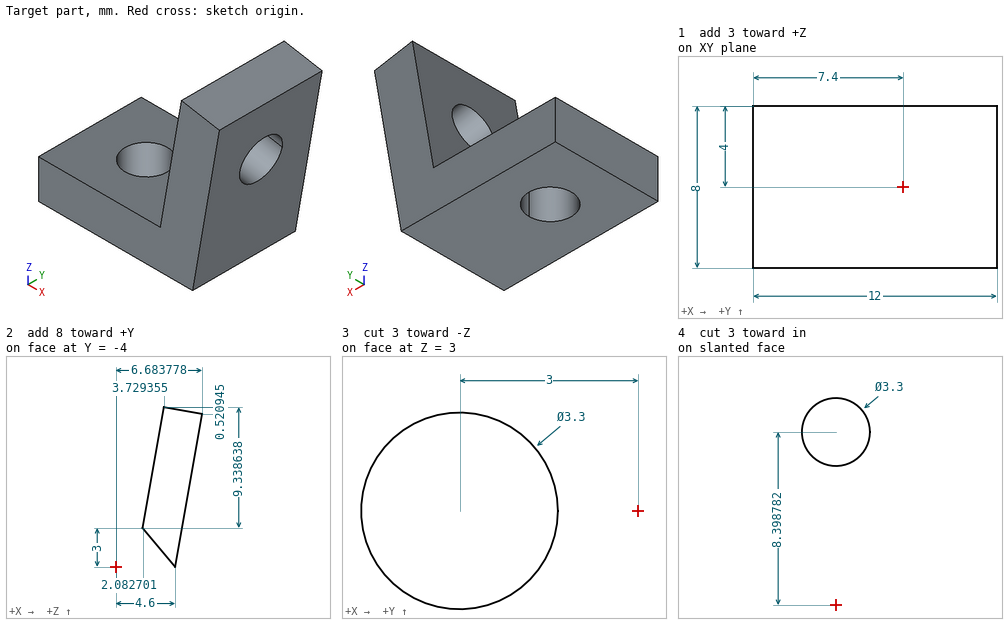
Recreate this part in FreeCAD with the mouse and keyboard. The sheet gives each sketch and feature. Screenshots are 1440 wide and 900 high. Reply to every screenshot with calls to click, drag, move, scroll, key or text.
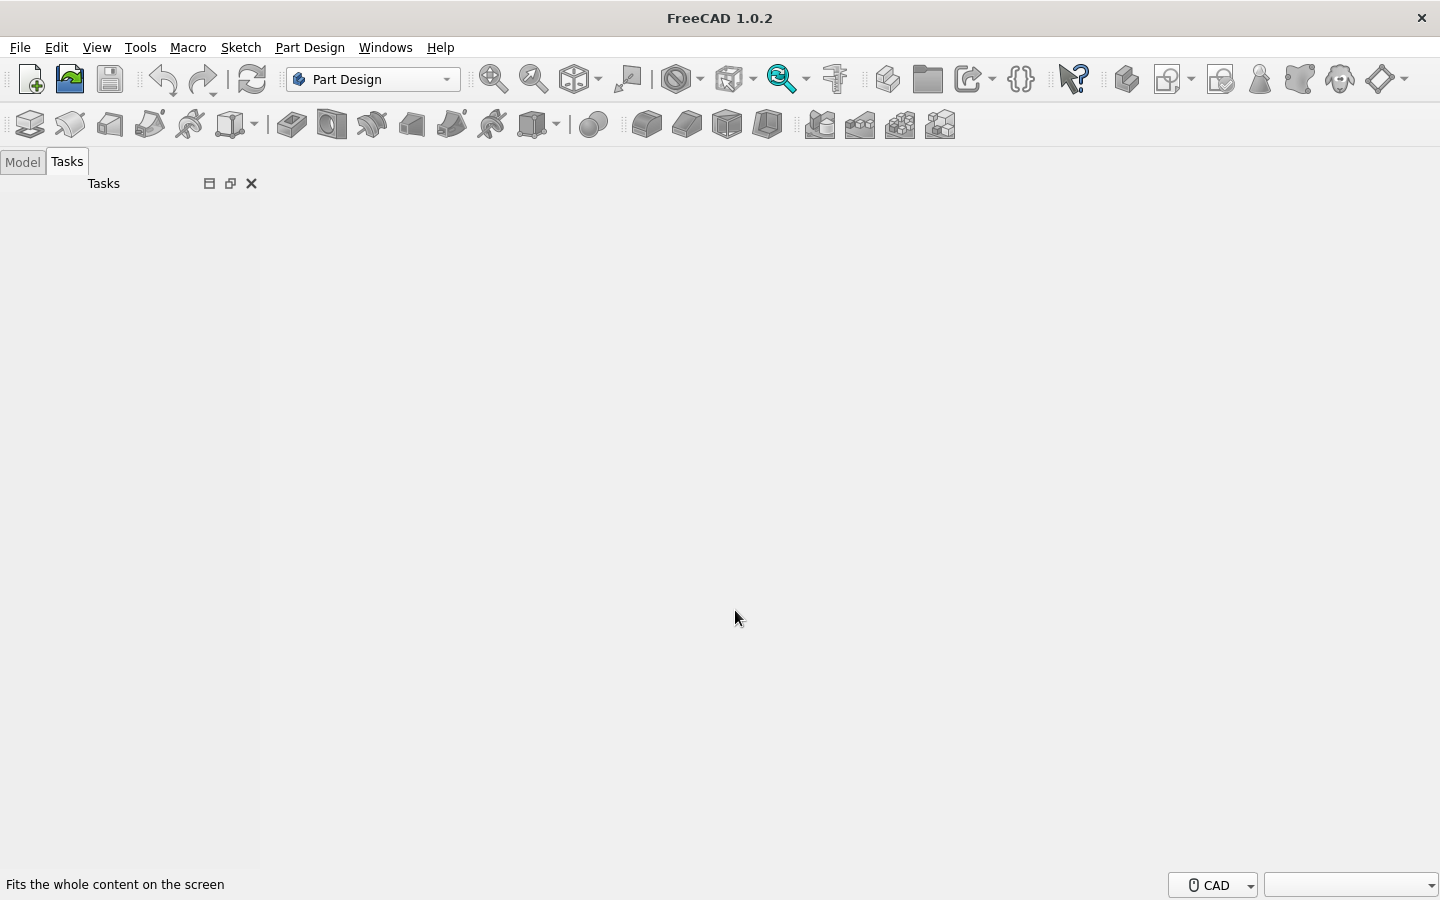
key(ctrl+n)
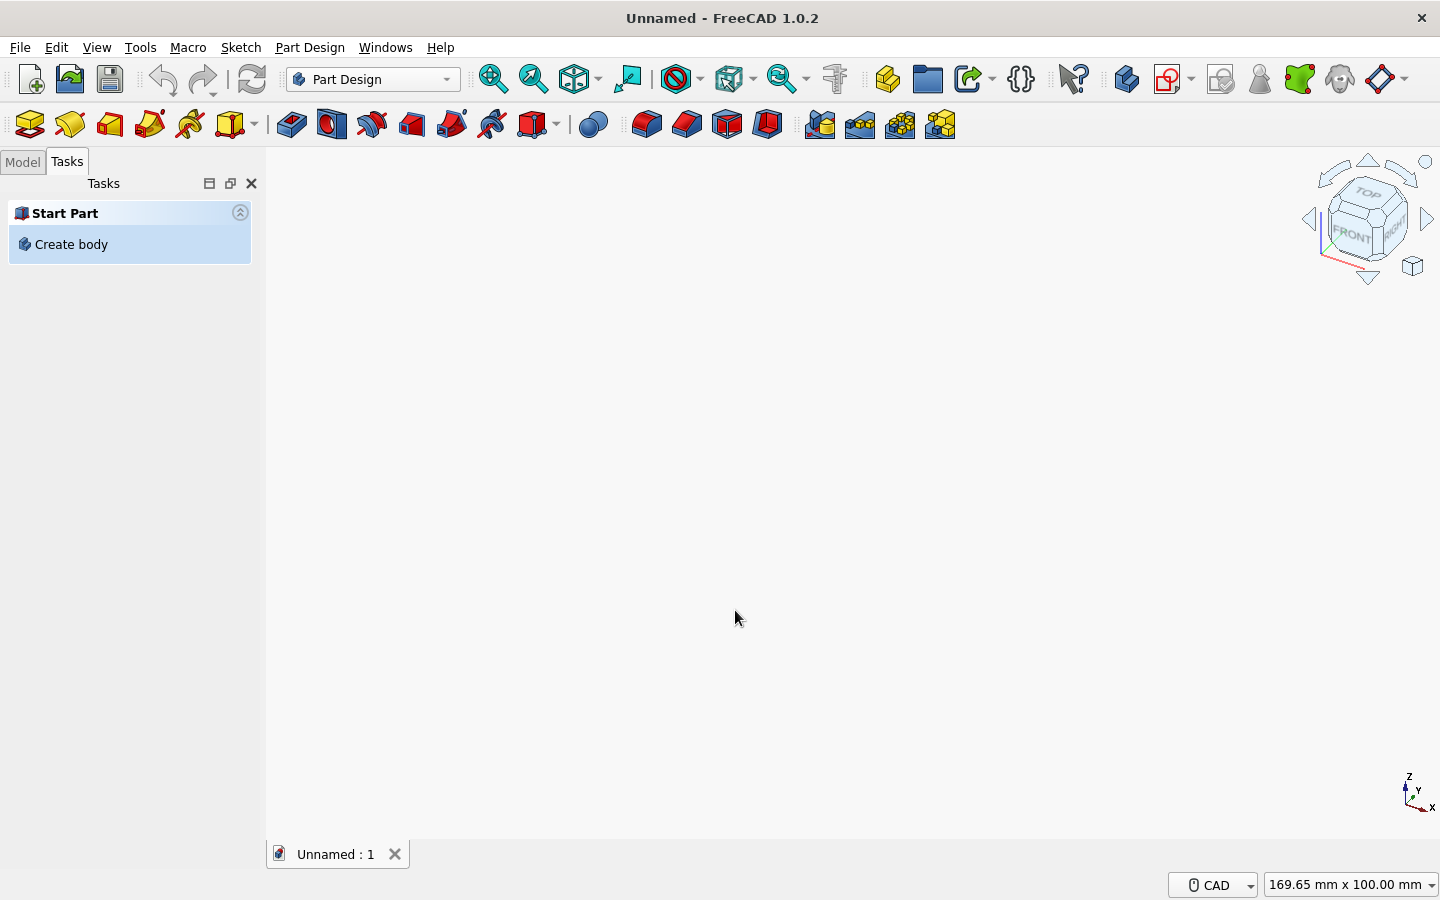
click(1168, 80)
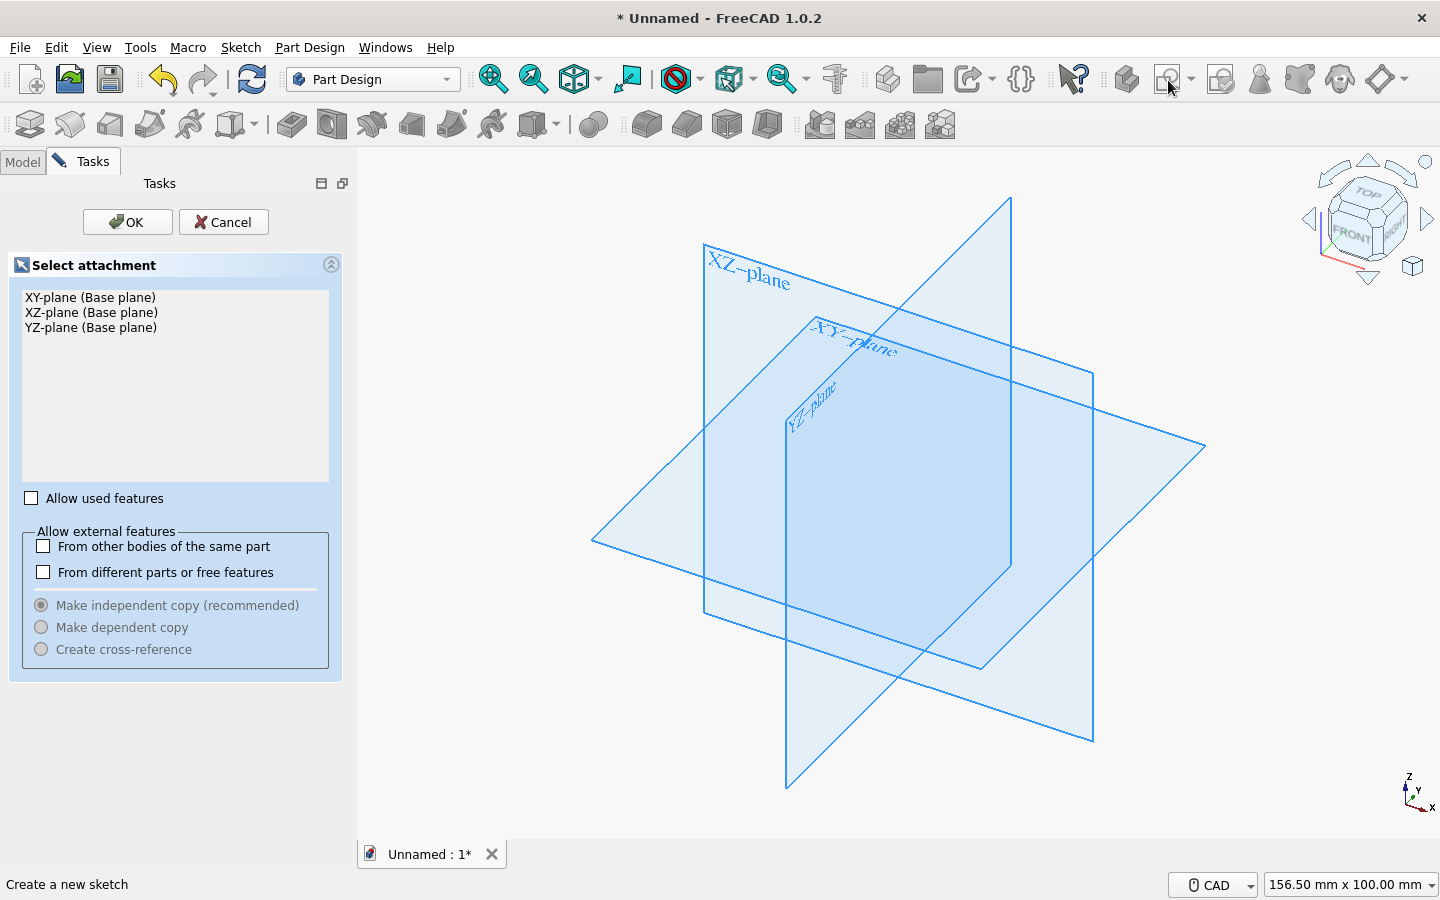
click(82, 298)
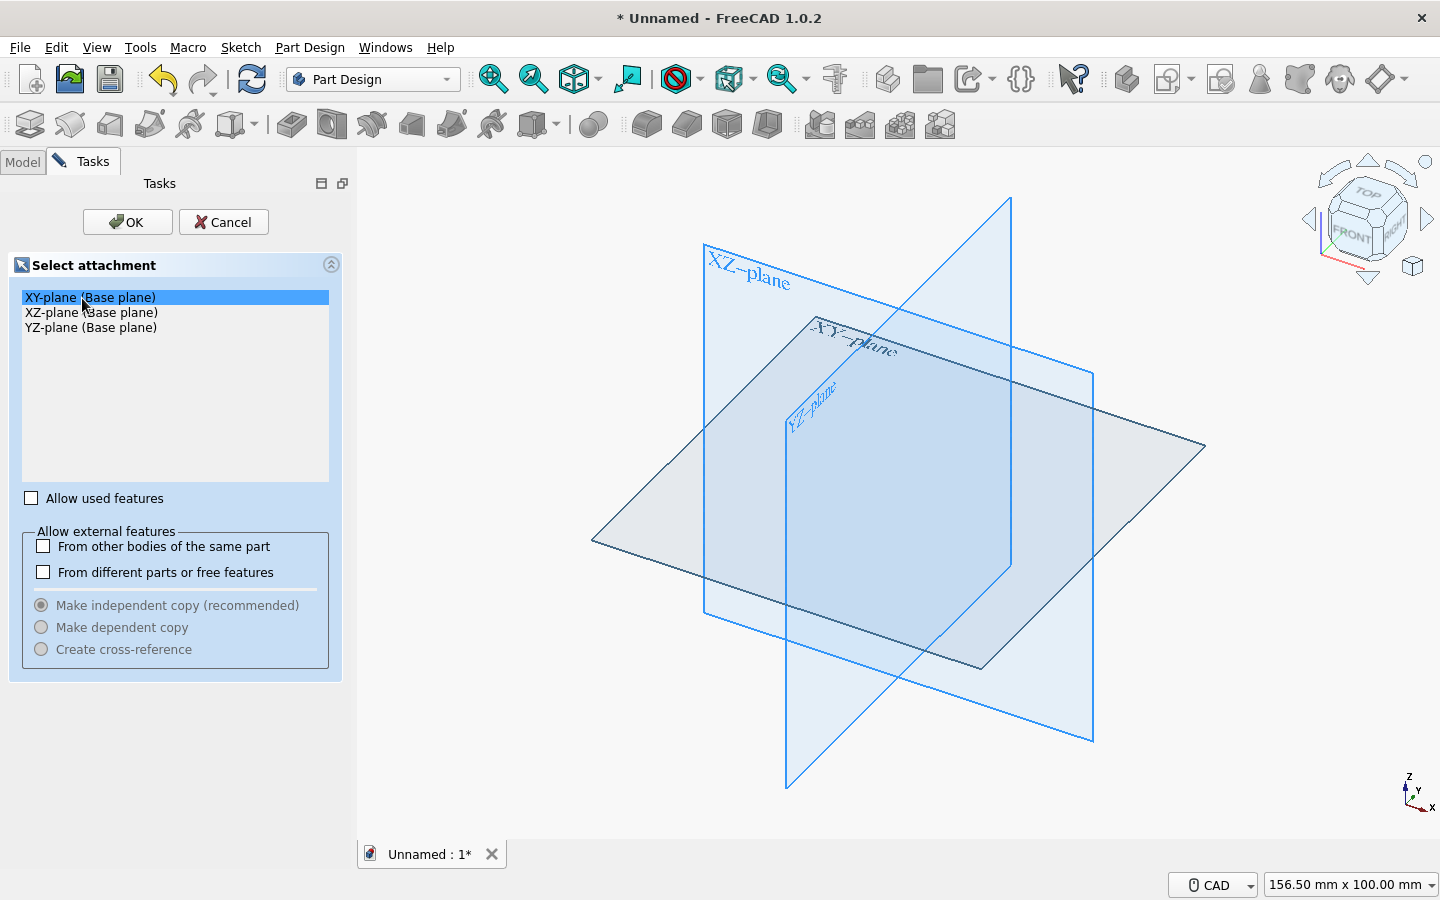
click(128, 222)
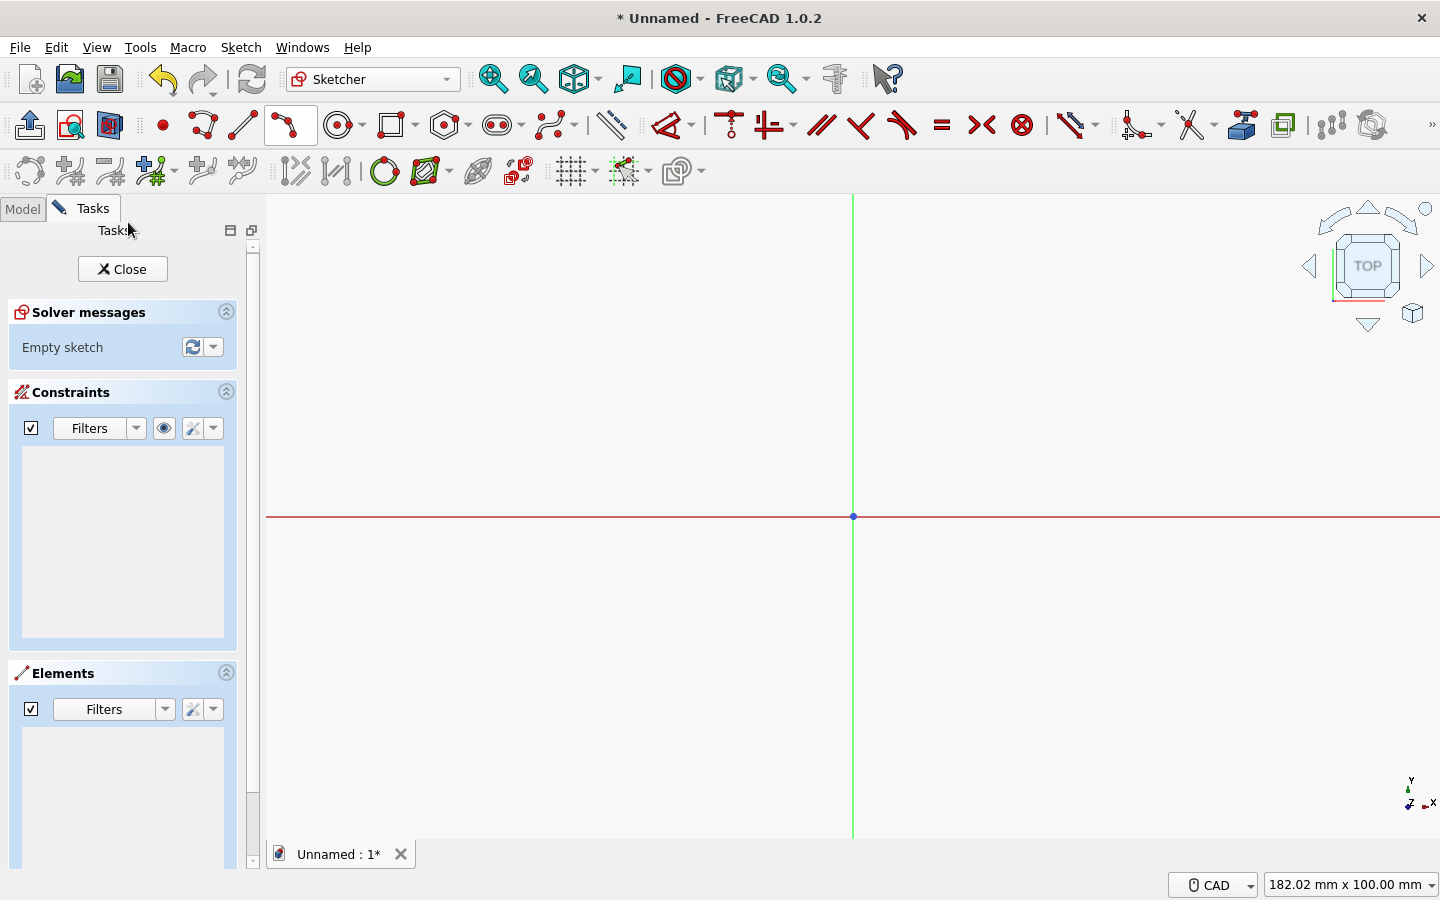
scroll(853, 516, up, 10)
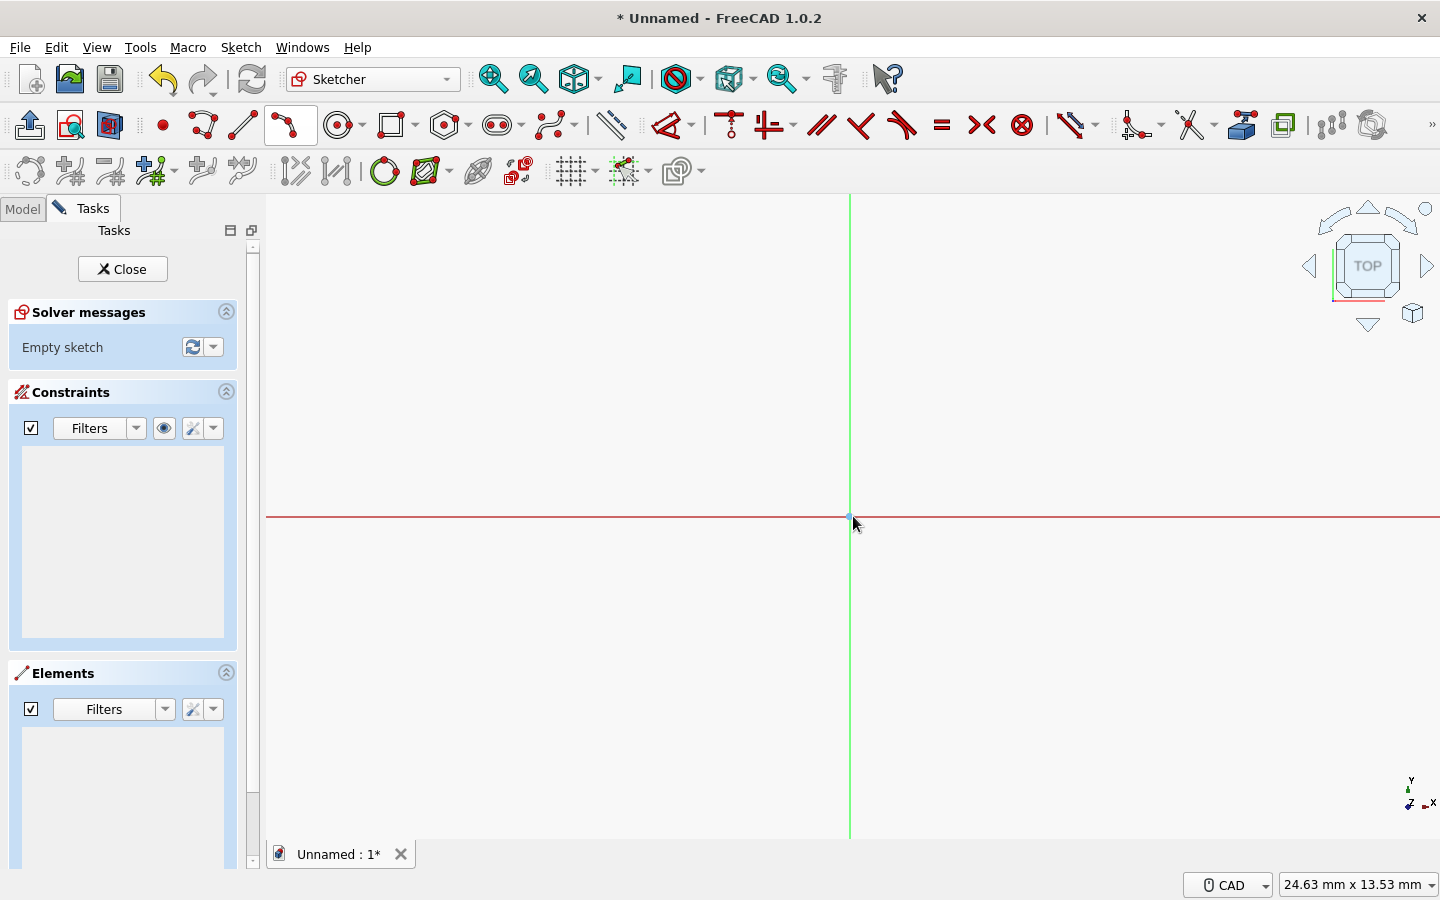
key(g)
key(r)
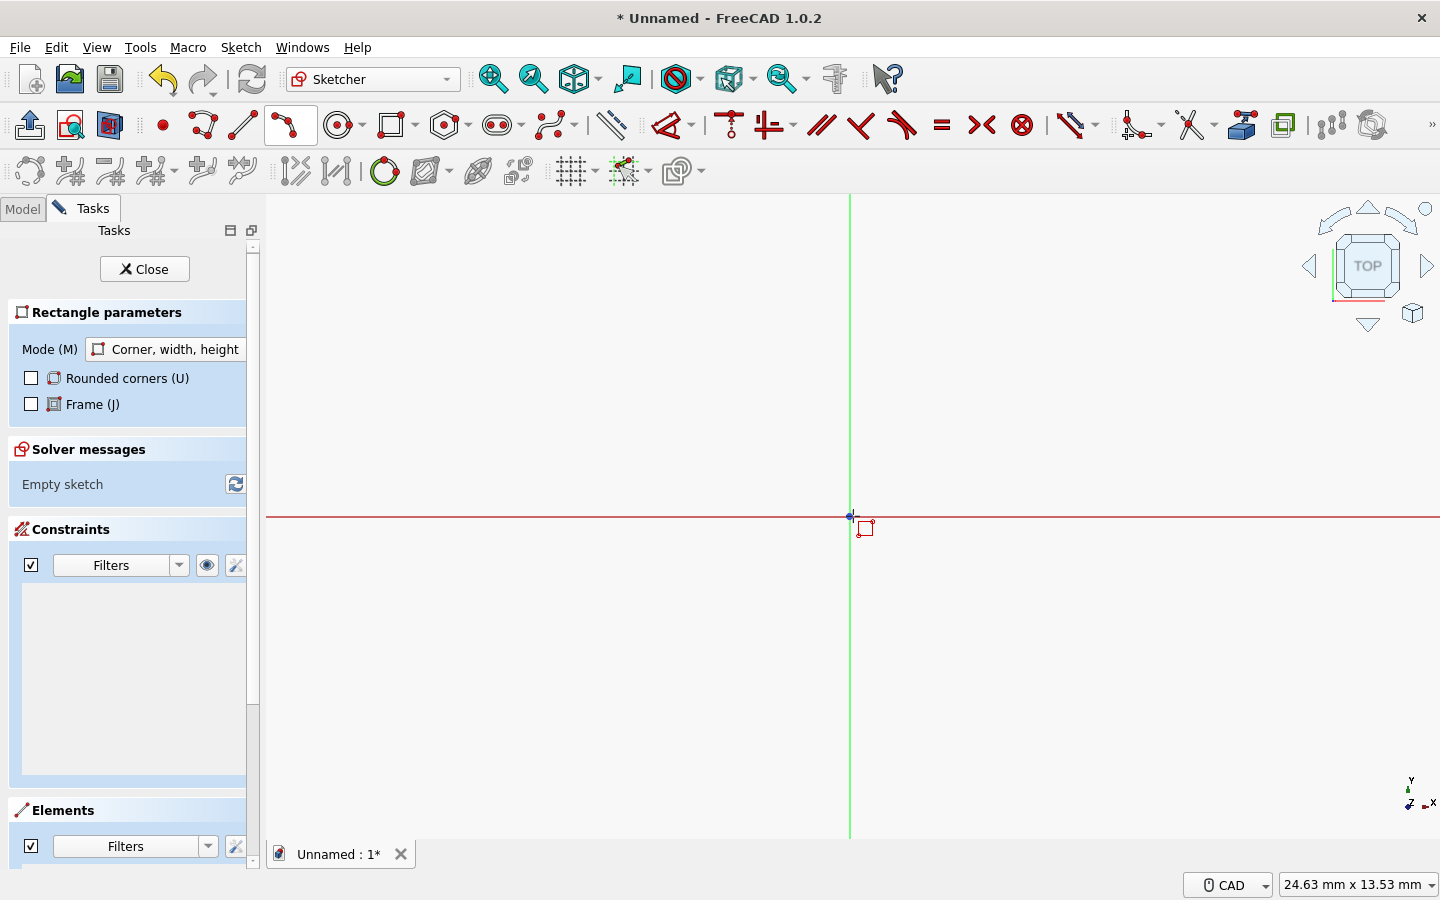
click(497, 326)
click(1069, 707)
key(Escape)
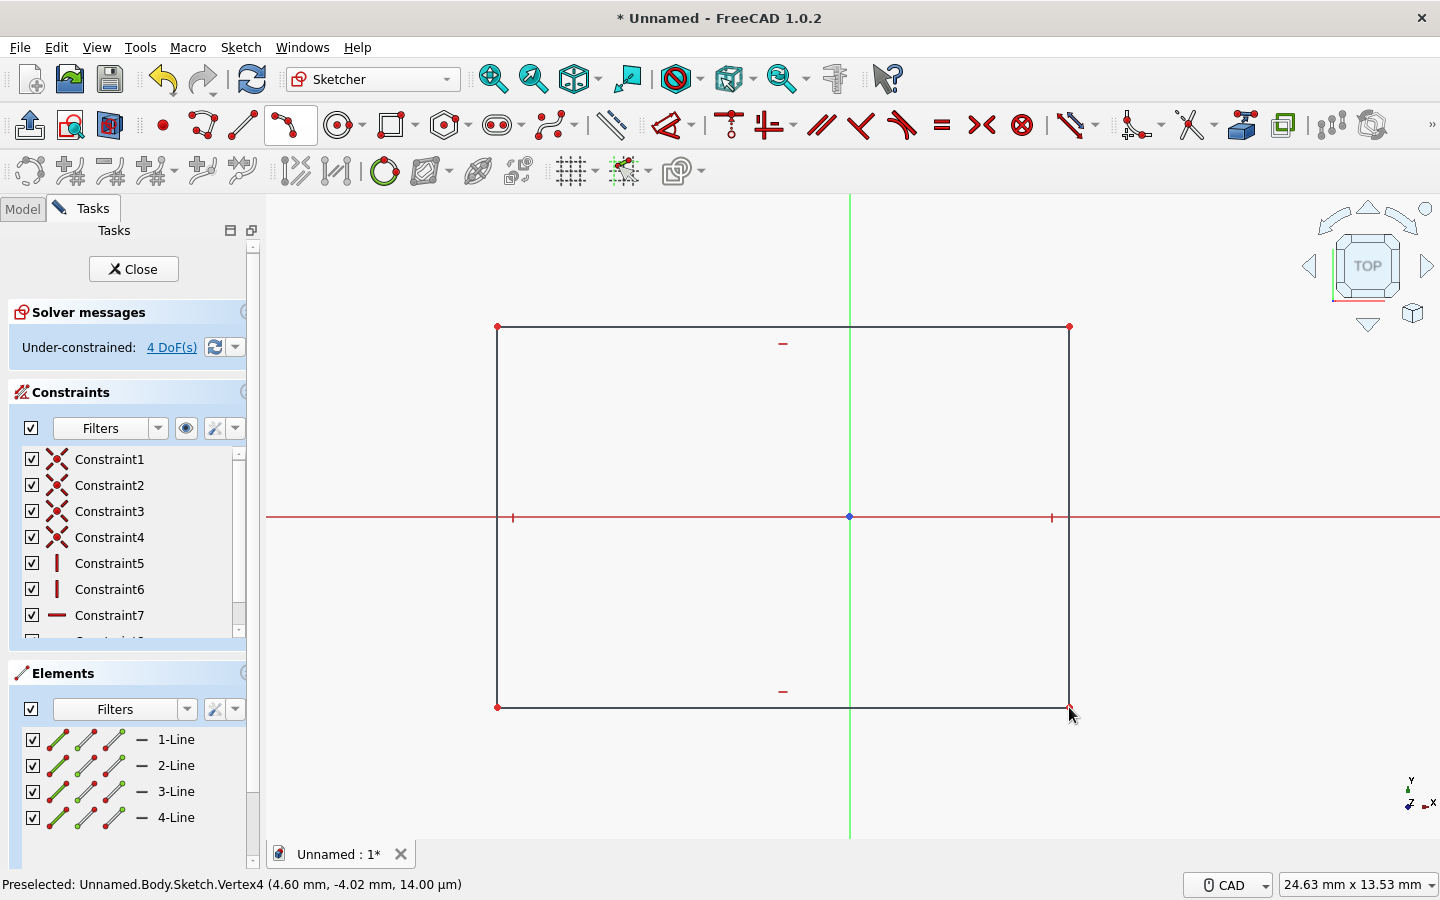
key(d)